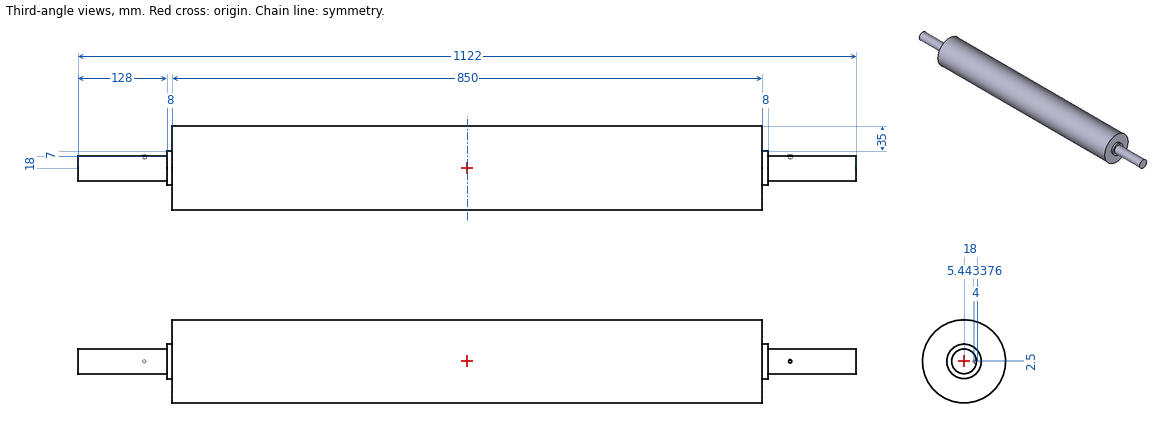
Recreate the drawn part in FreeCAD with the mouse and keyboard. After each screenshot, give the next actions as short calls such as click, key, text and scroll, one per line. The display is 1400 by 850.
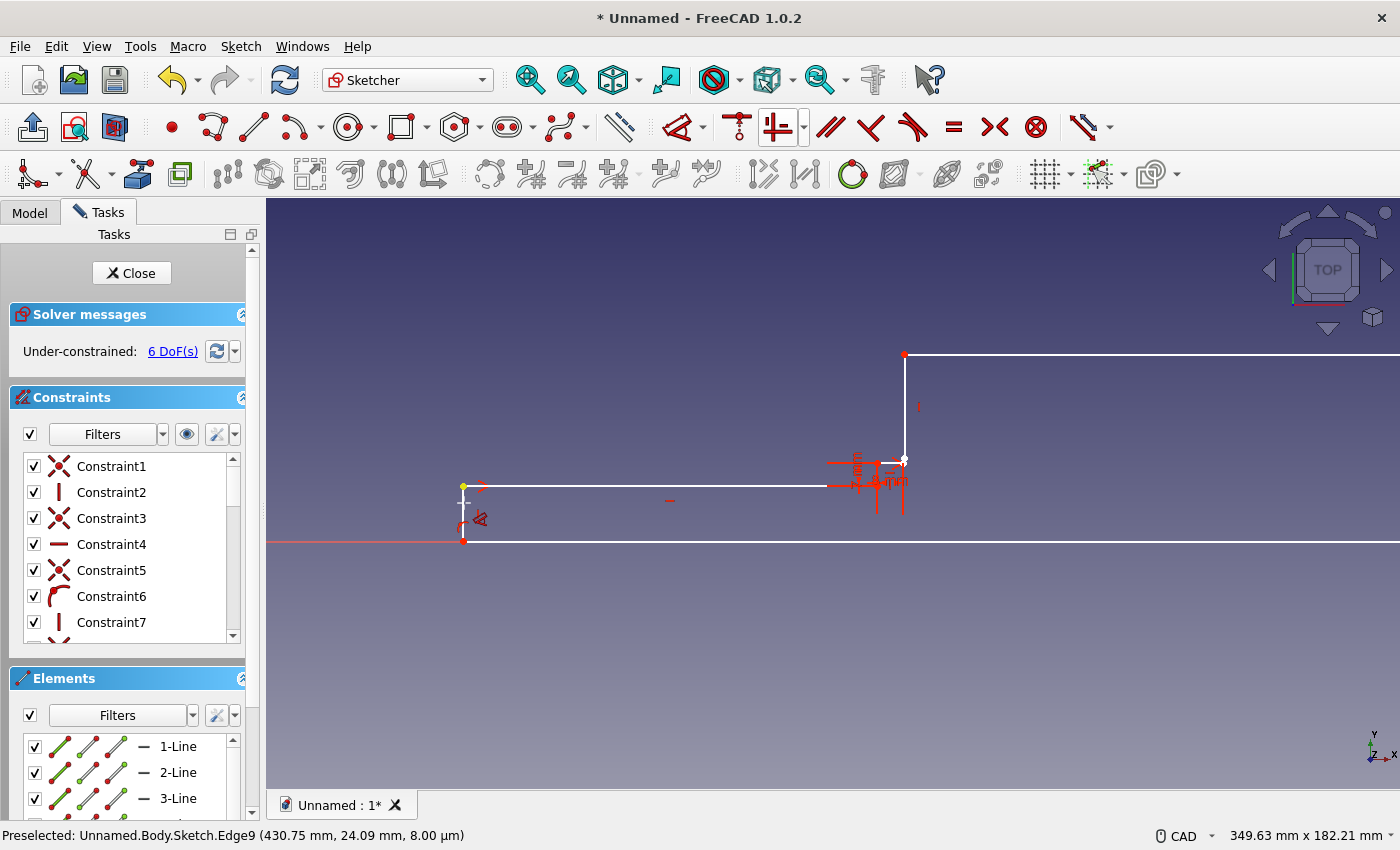
click(463, 503)
click(429, 514)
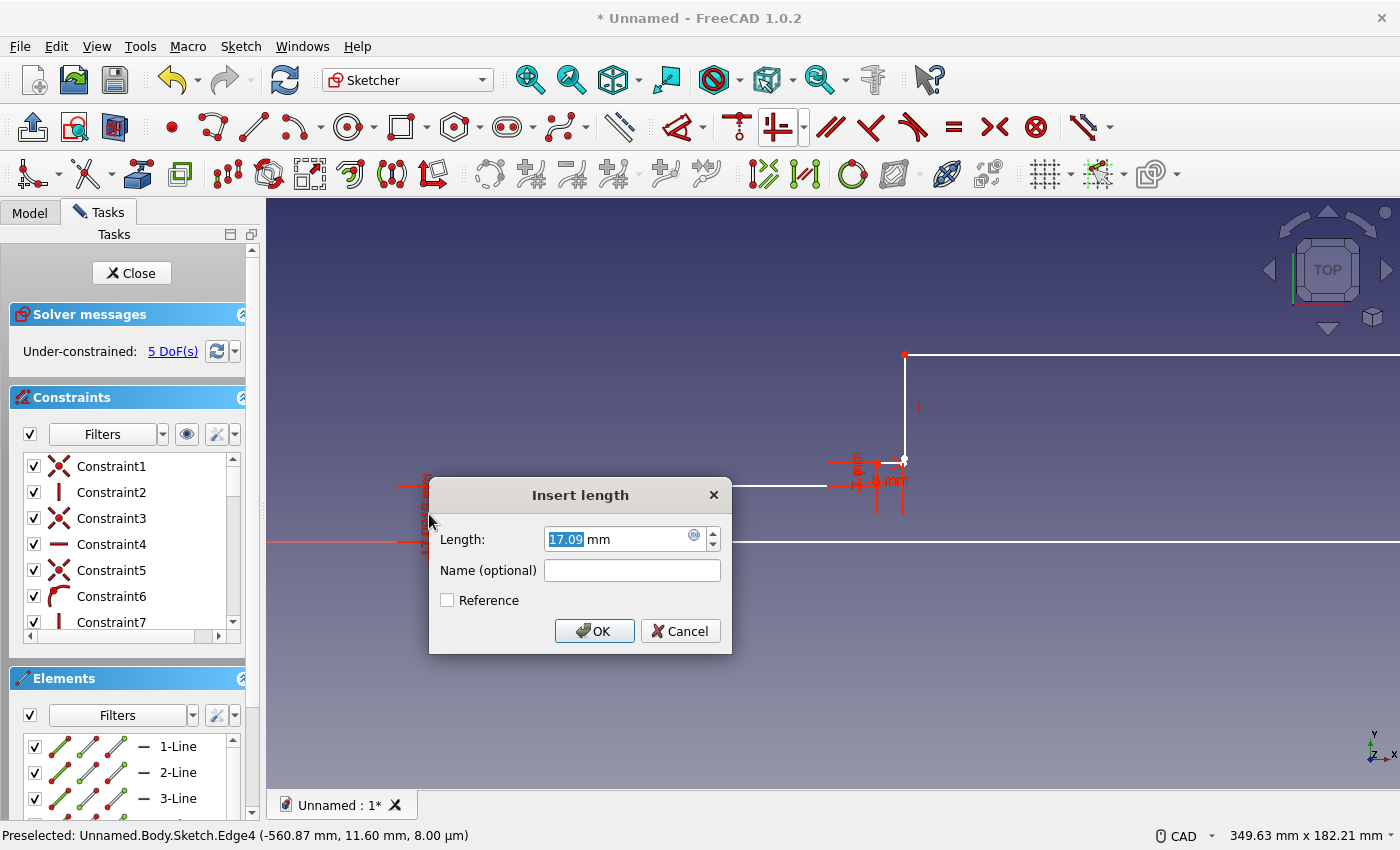
text(18)
key(Return)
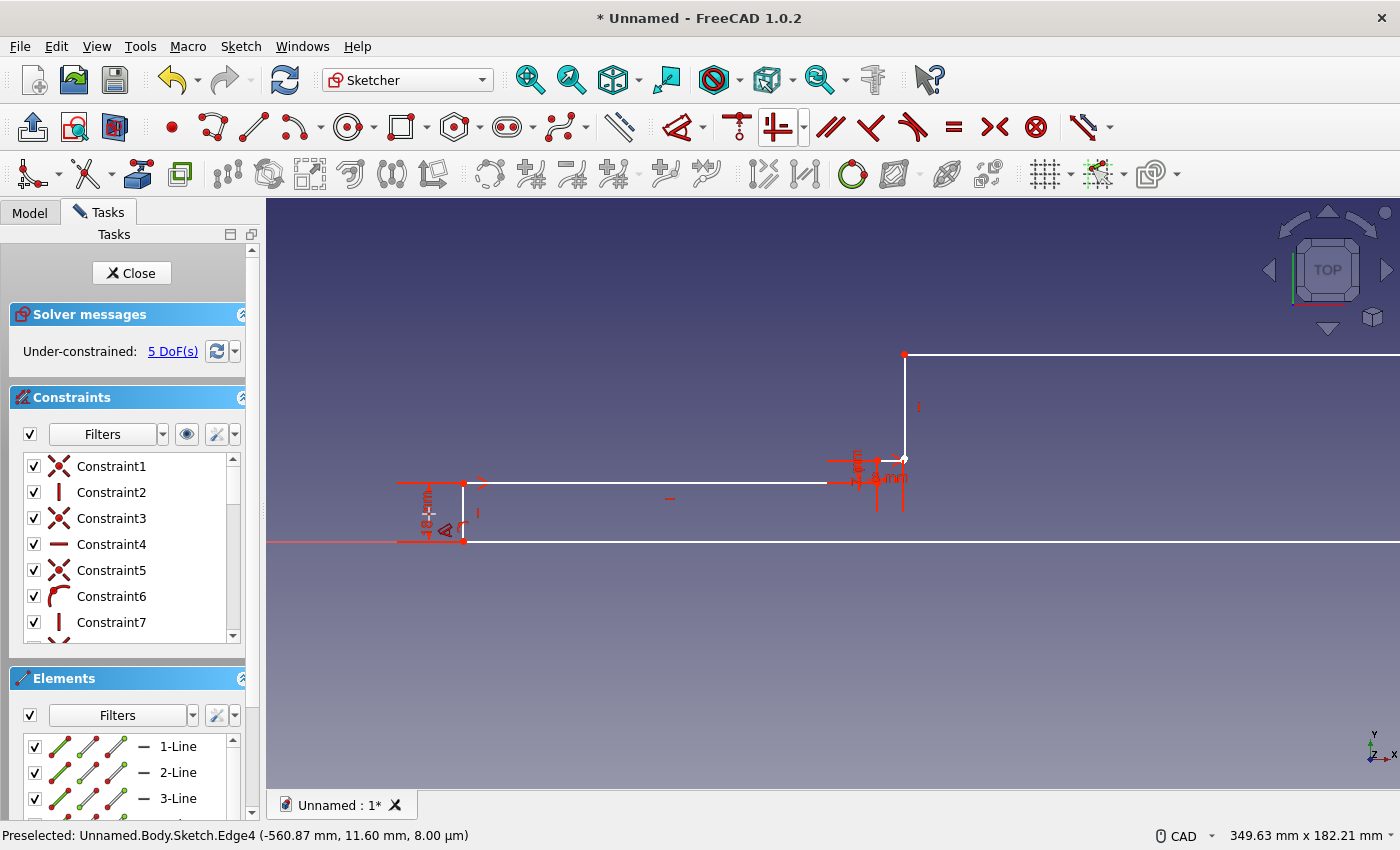
scroll(464, 503, down, 9)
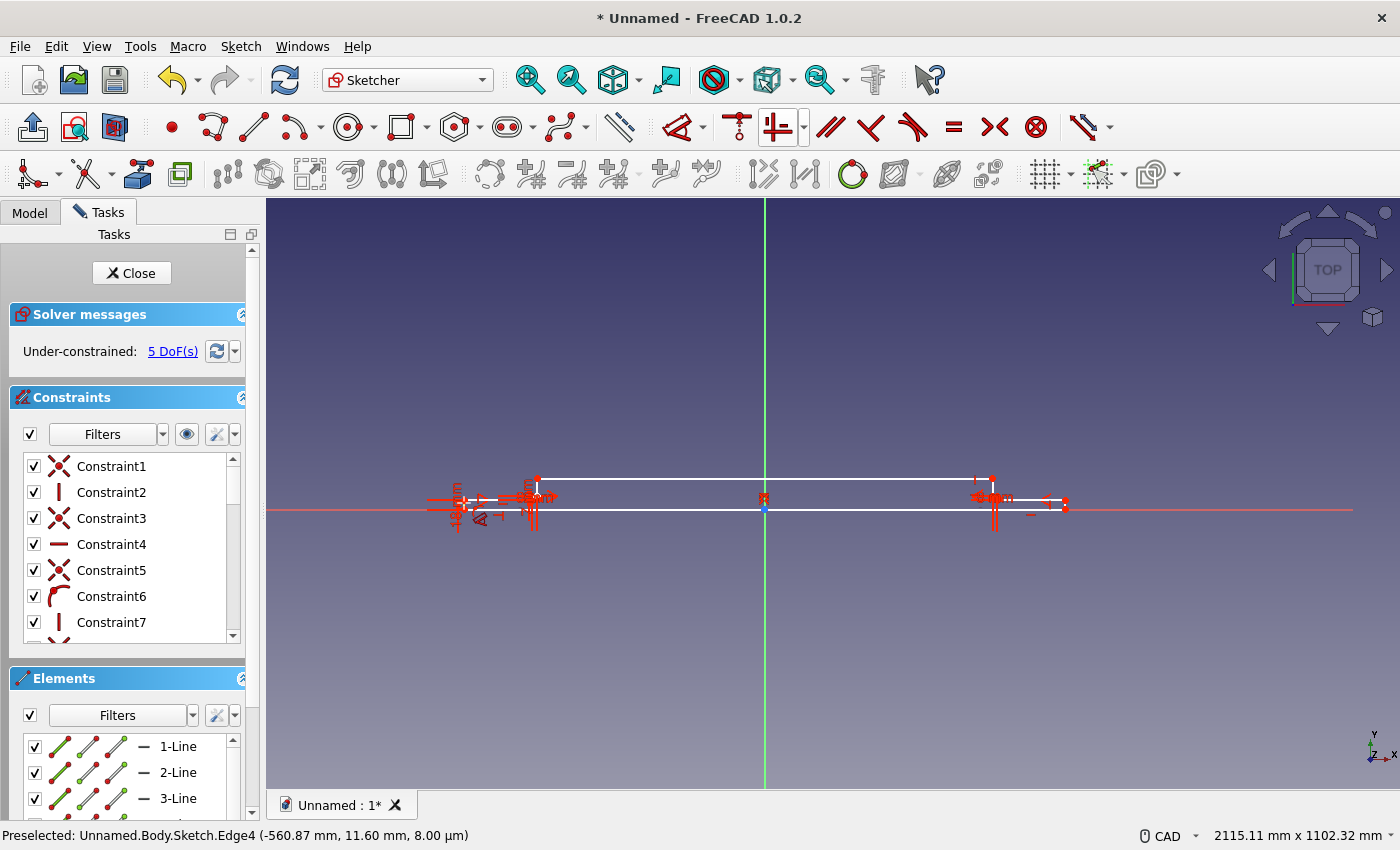
scroll(993, 491, up, 5)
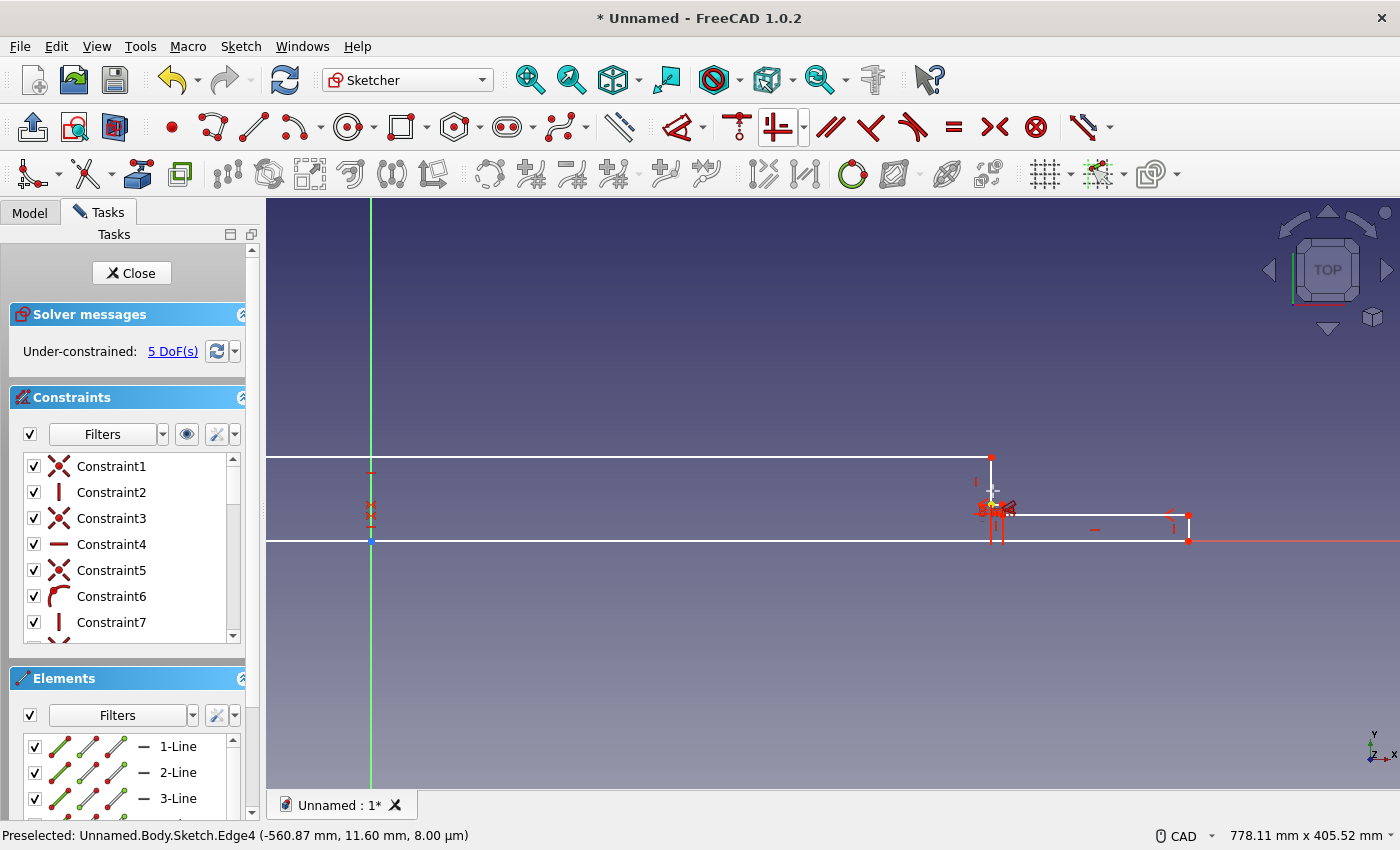
click(991, 491)
click(1025, 481)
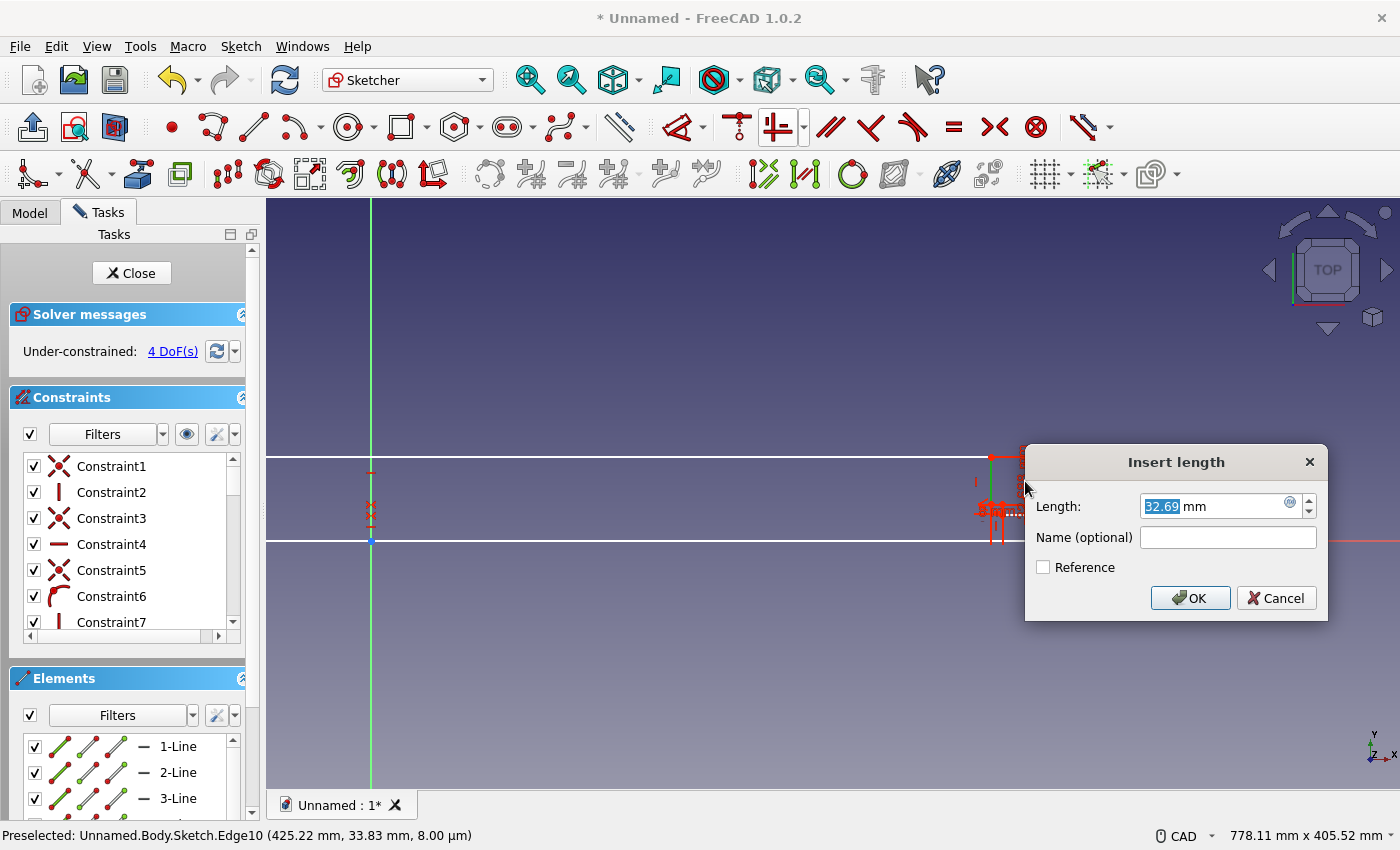
text(35)
key(Return)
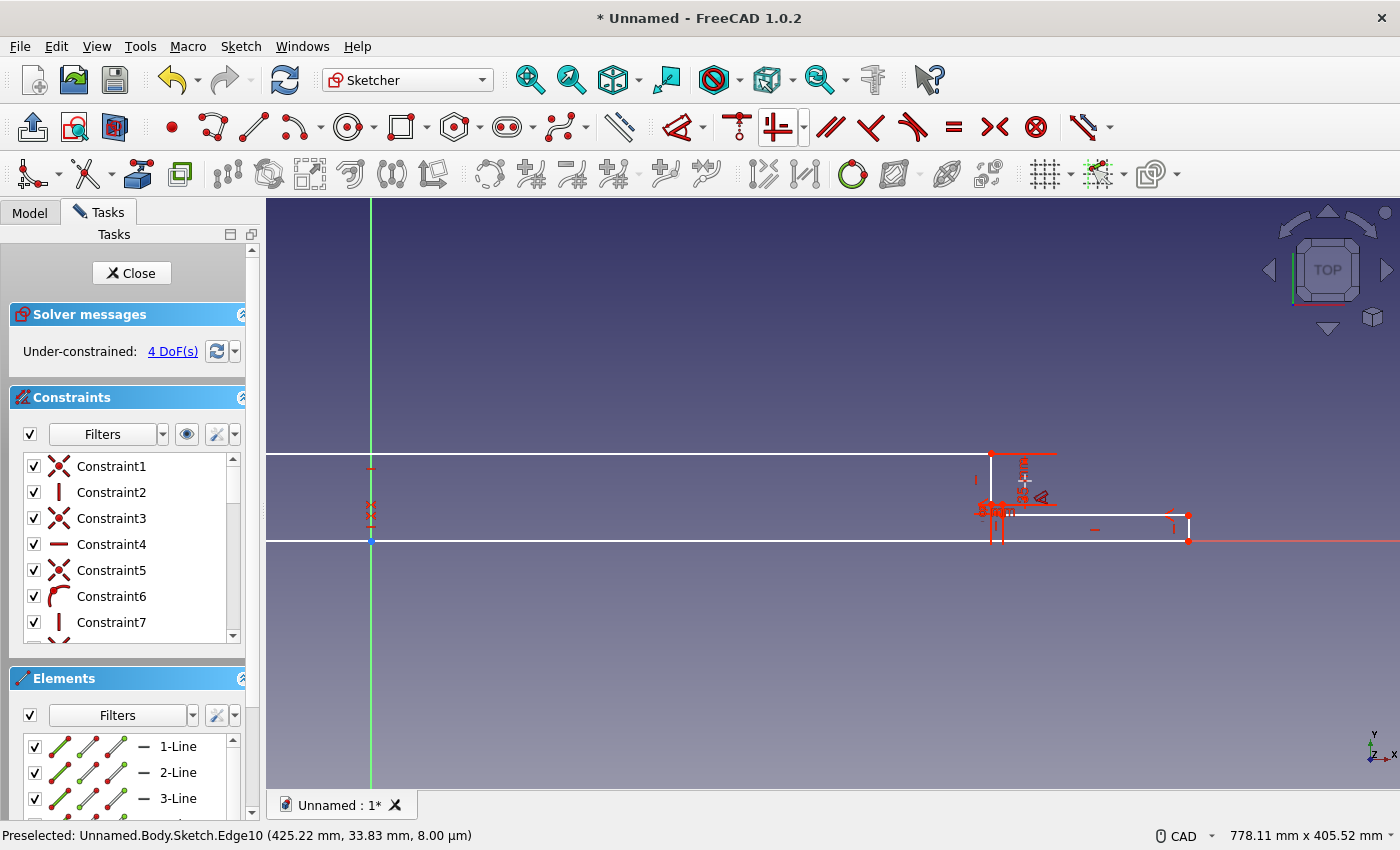
scroll(993, 491, down, 5)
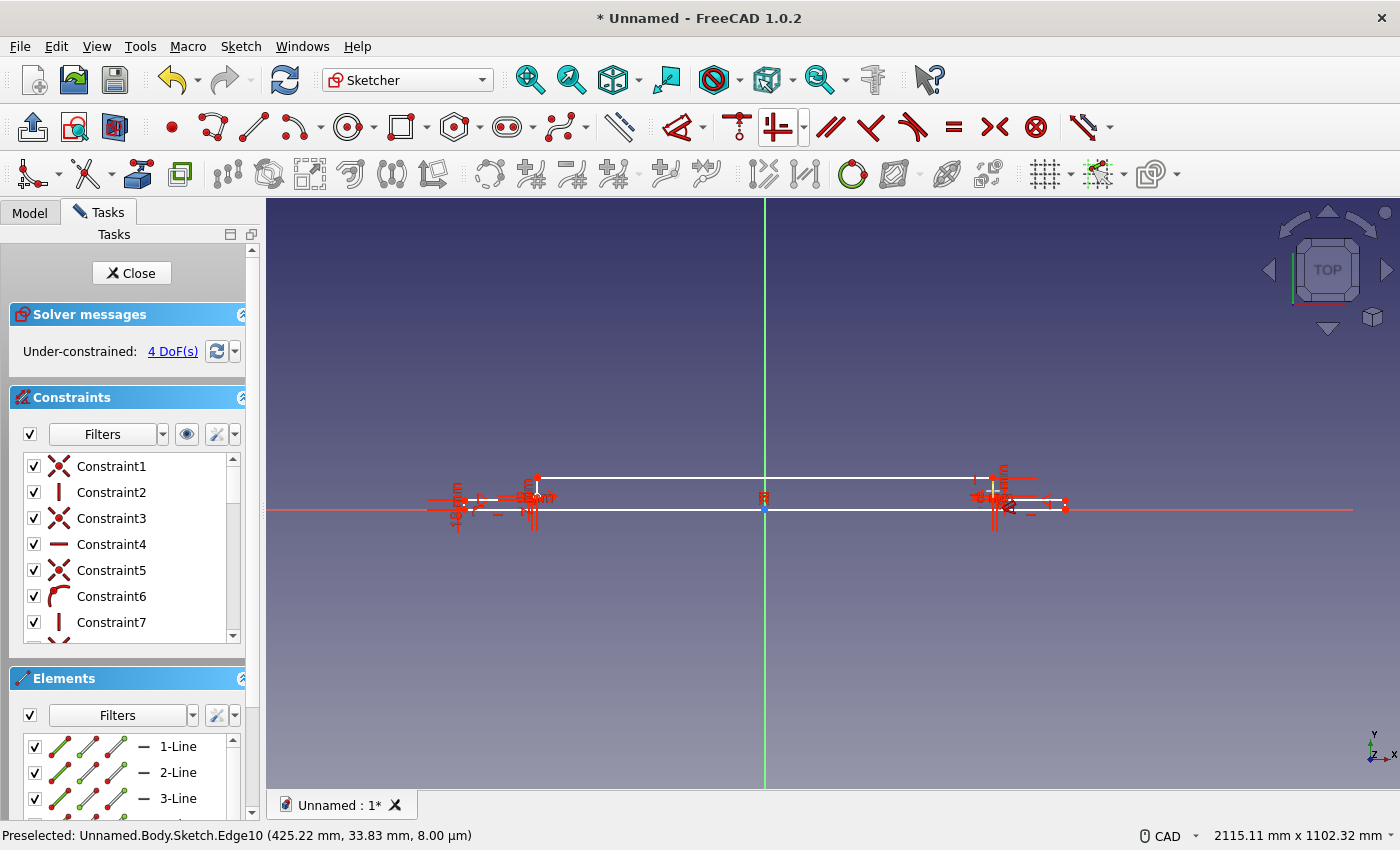
scroll(537, 483, up, 5)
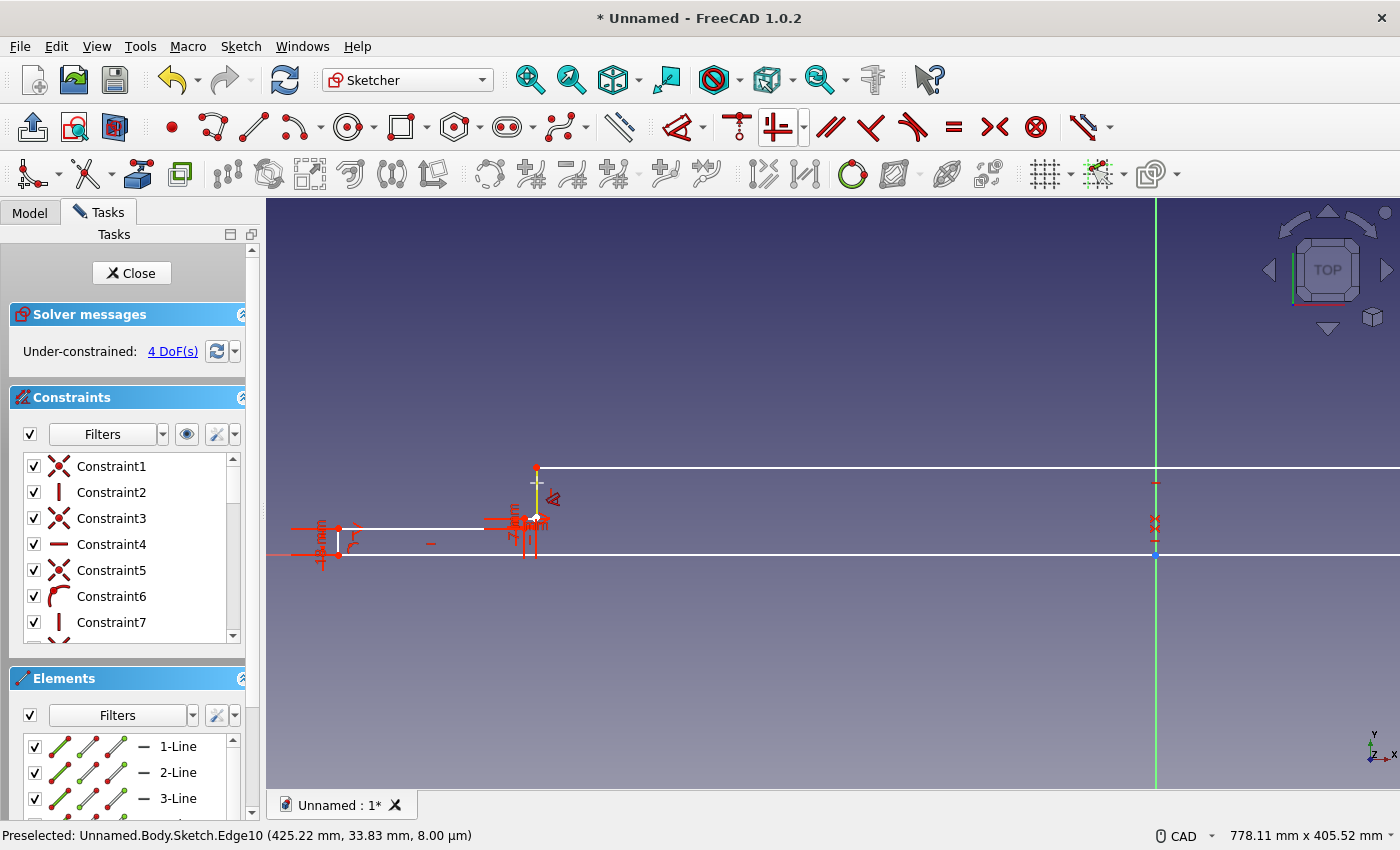
click(537, 483)
click(503, 493)